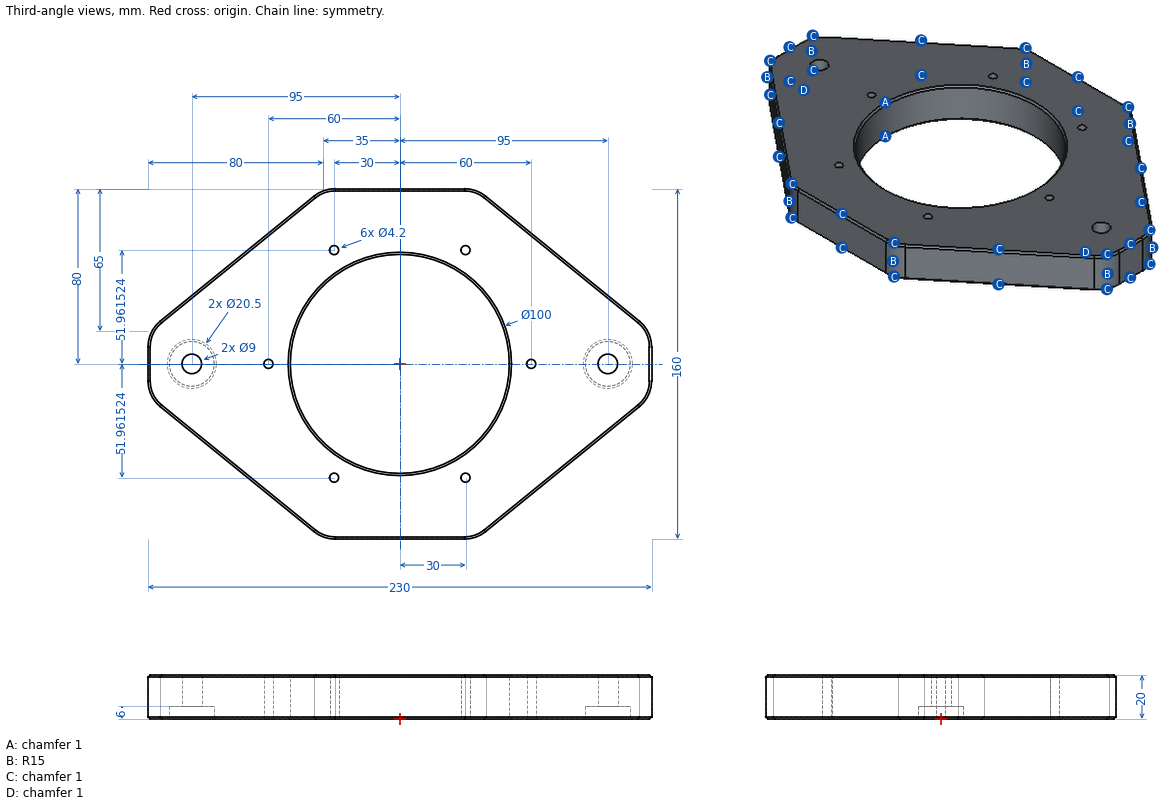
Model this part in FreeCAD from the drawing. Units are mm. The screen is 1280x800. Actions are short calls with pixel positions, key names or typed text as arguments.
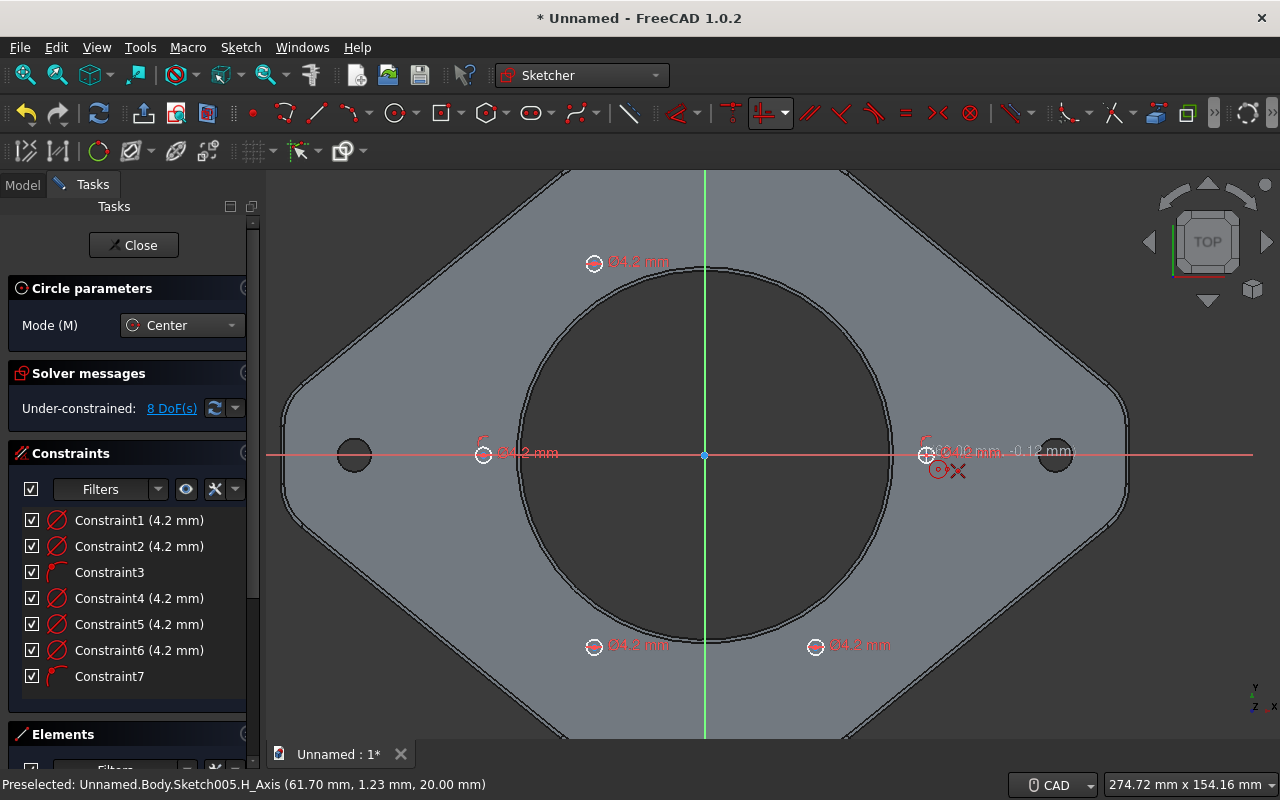
scroll(816, 263, up, 6)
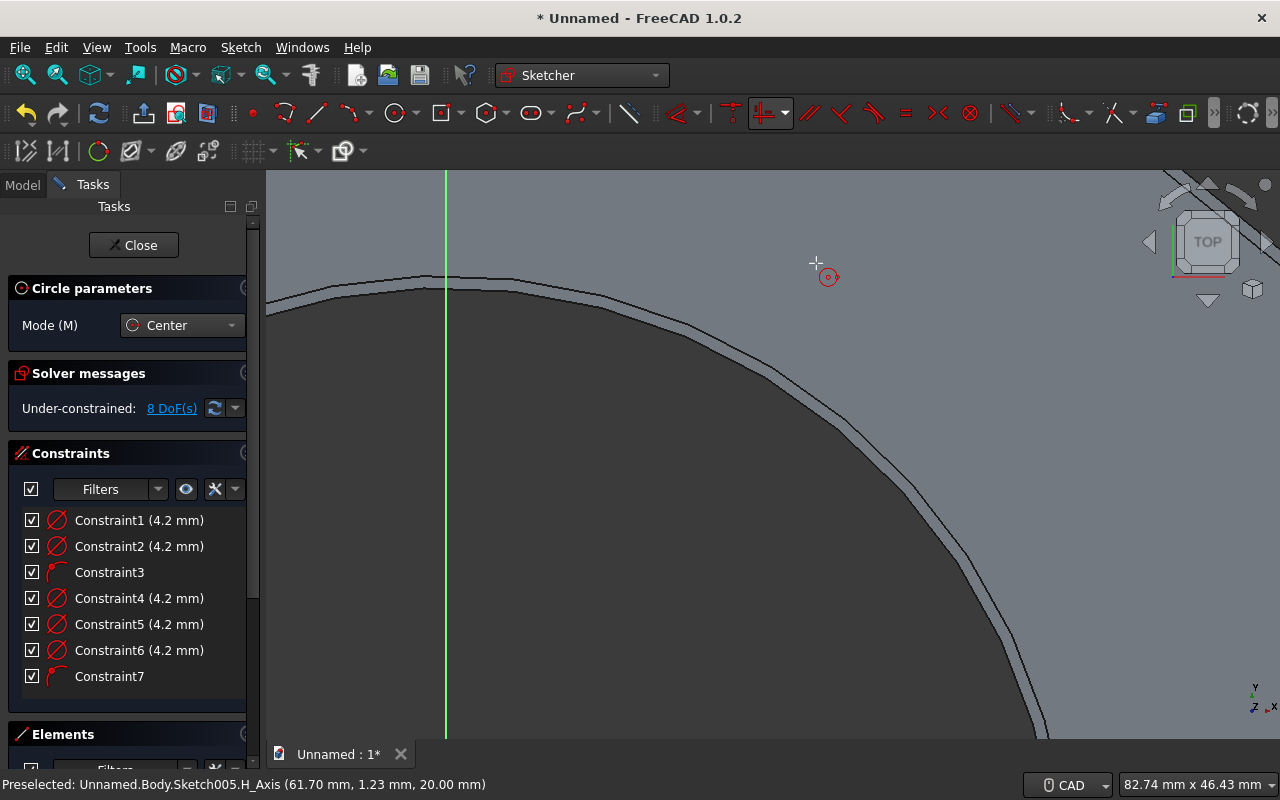
click(814, 264)
move(832, 246)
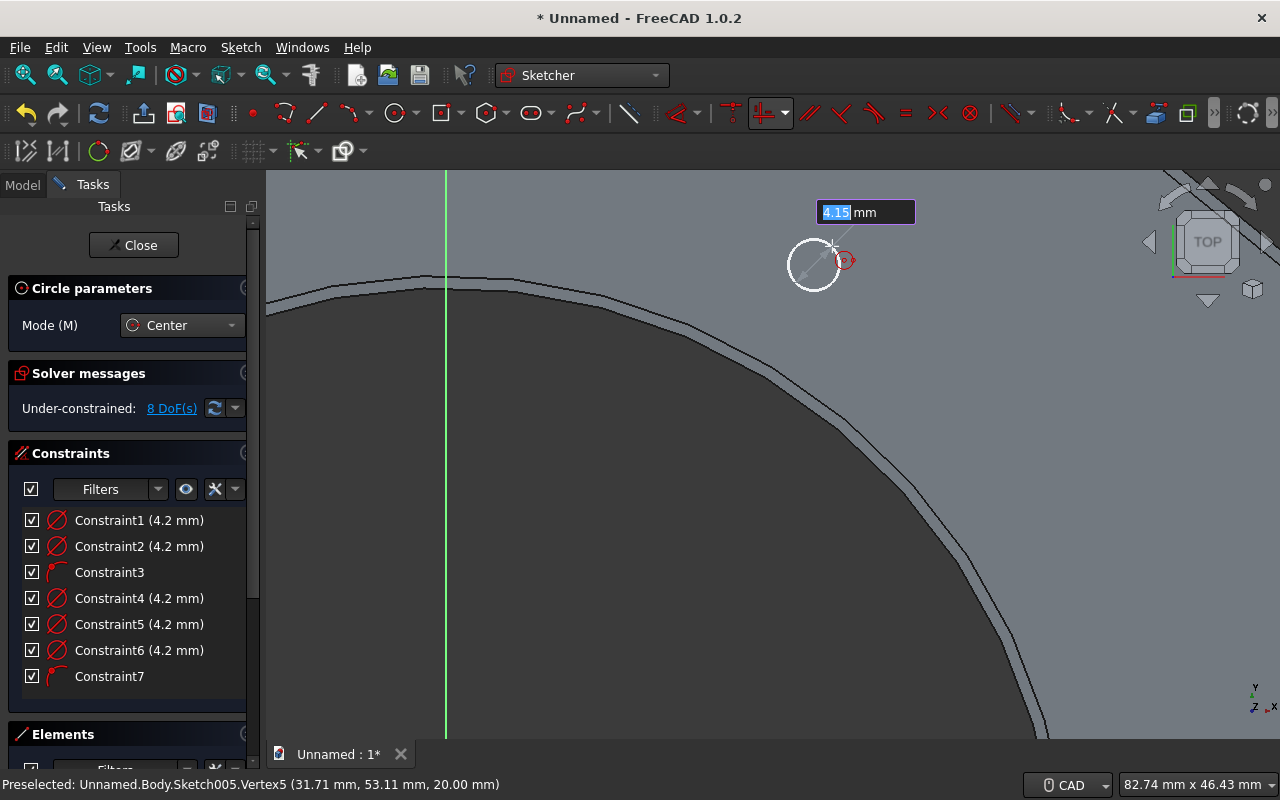
text(4.2)
key(Return)
key(Escape)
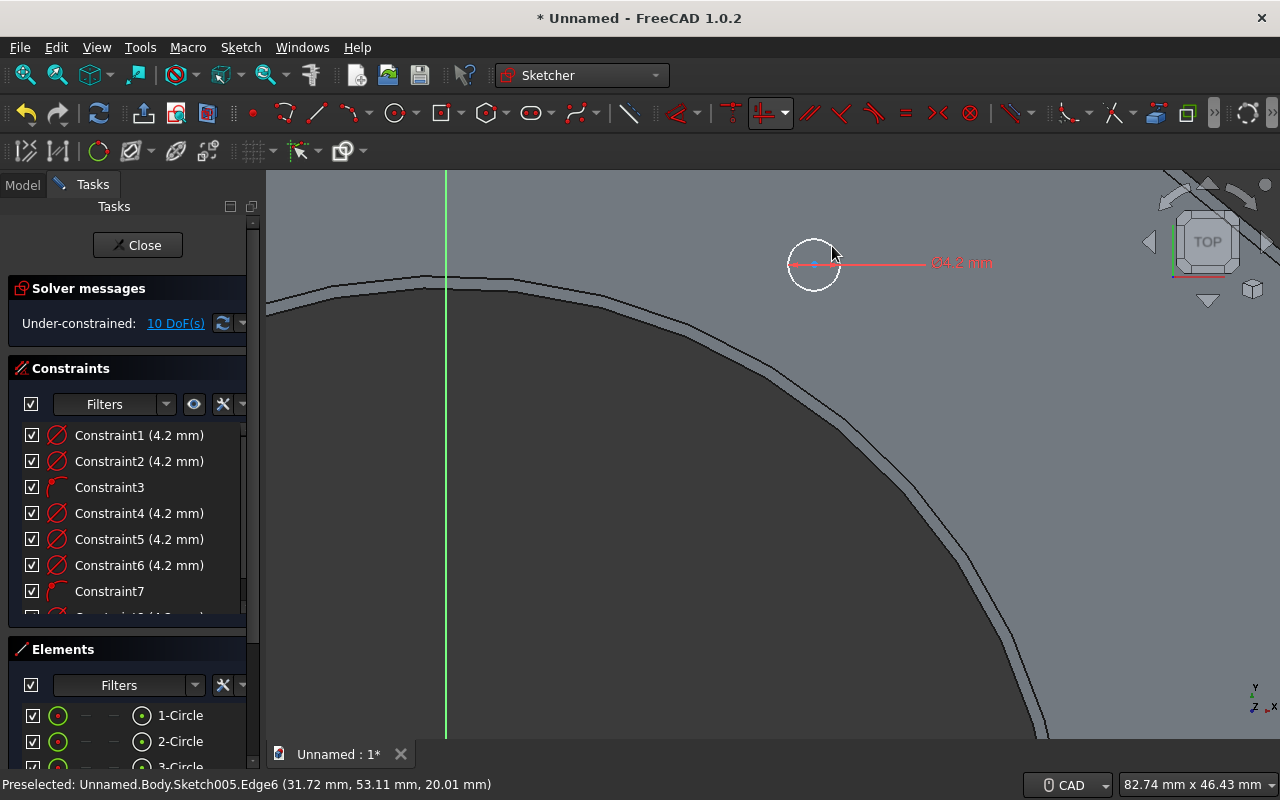
scroll(816, 262, down, 6)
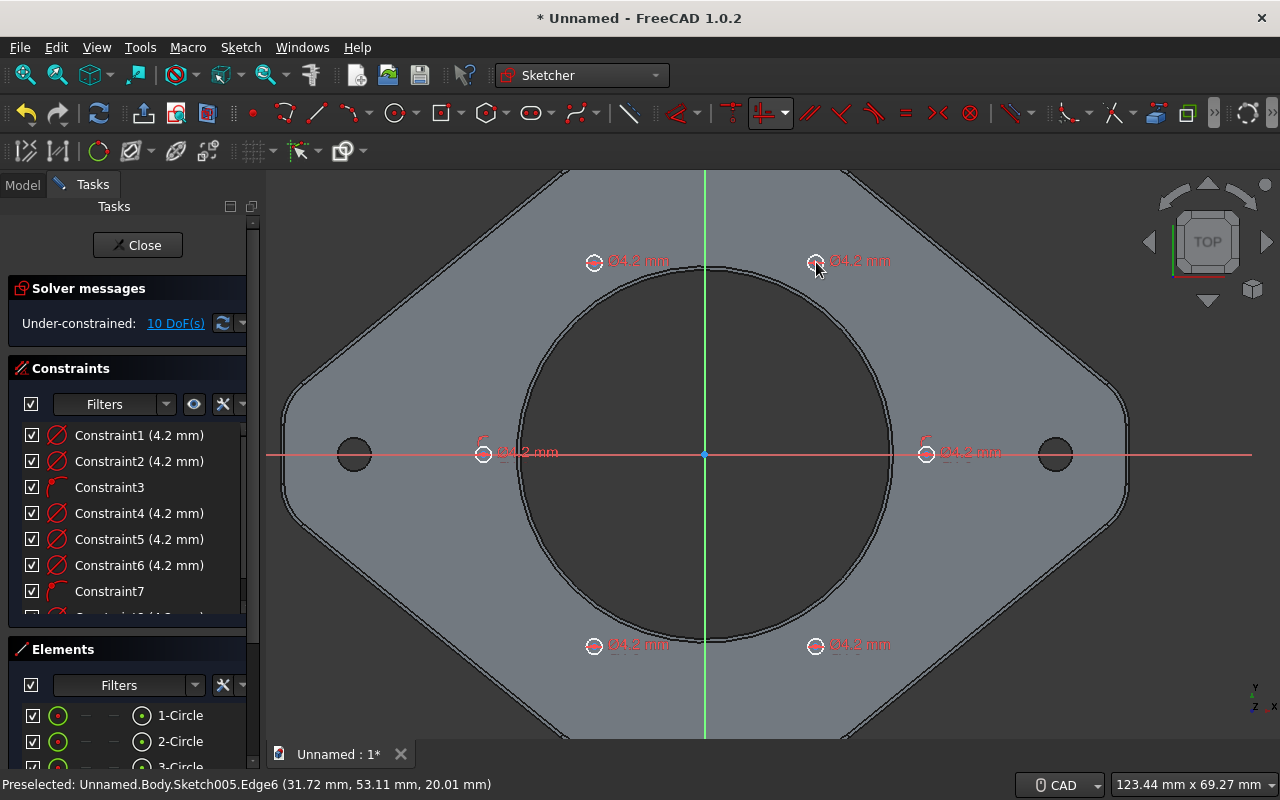
click(594, 263)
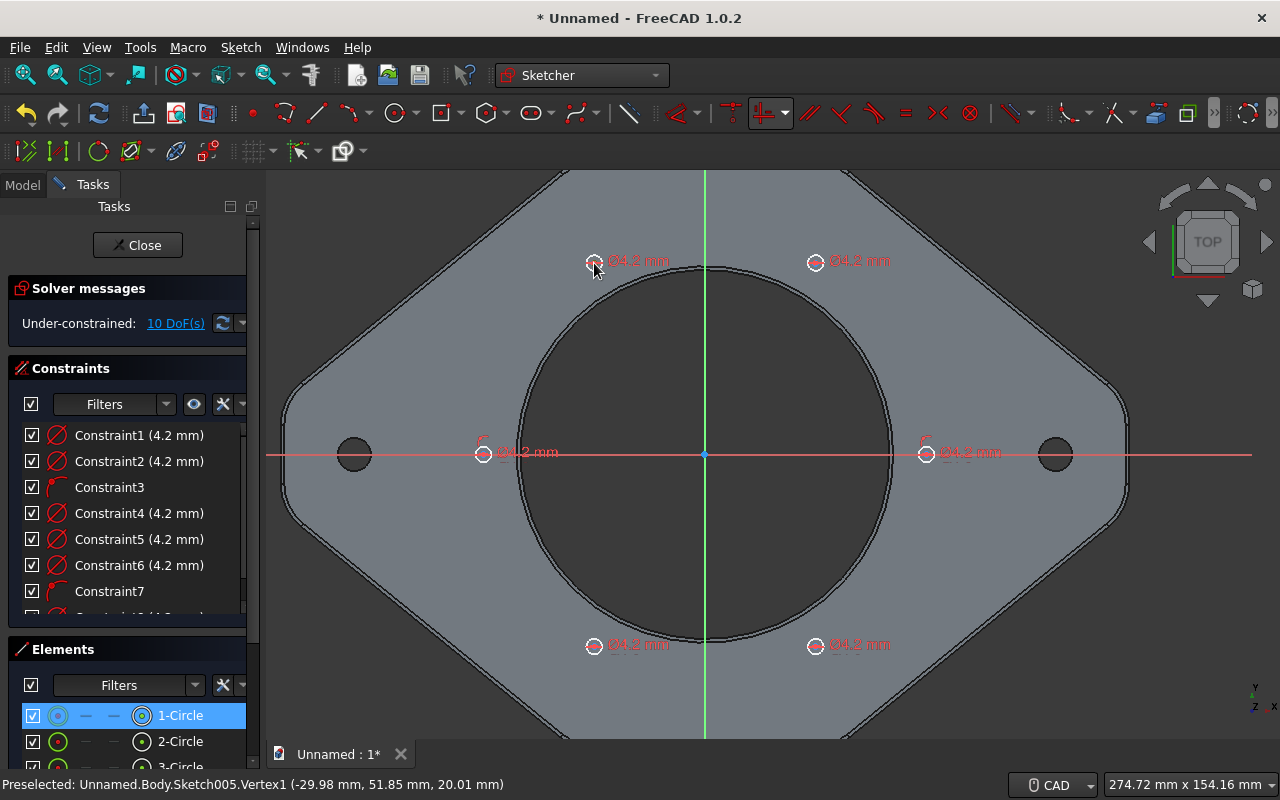
click(594, 647)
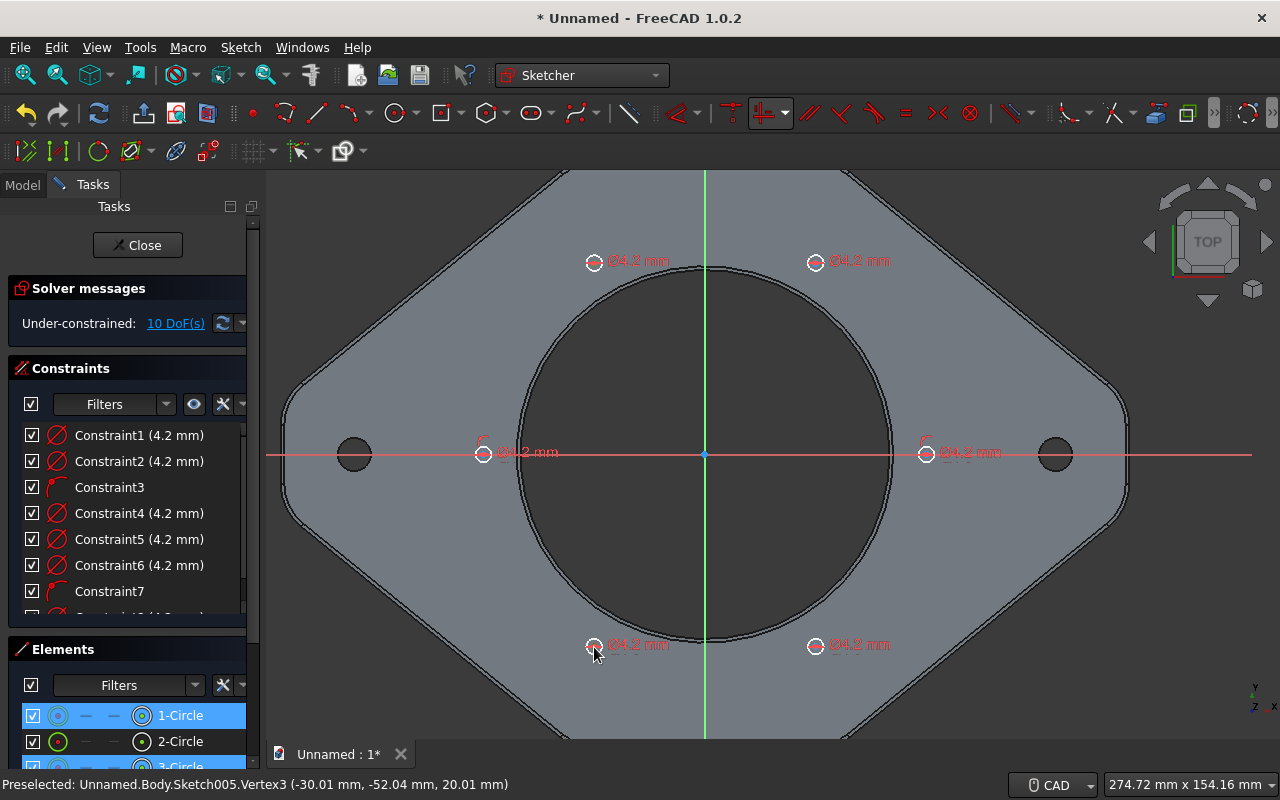
click(788, 114)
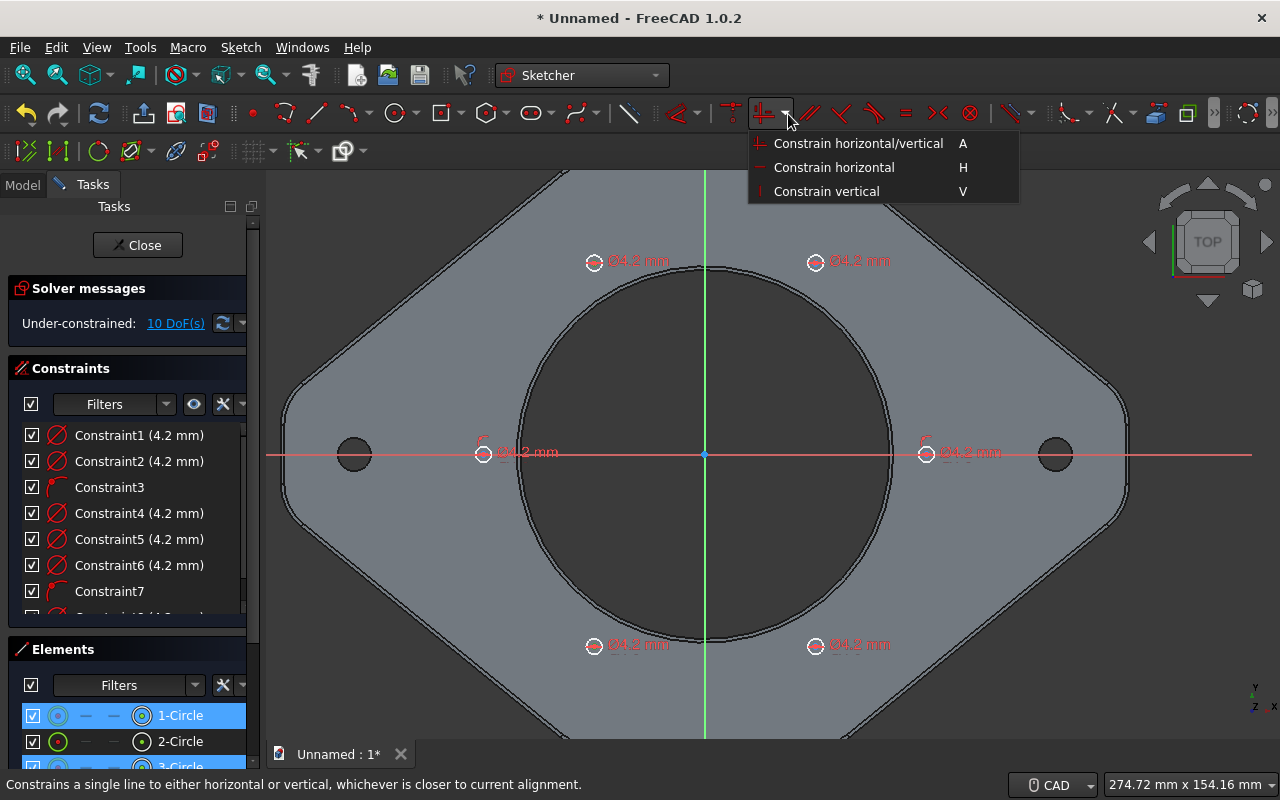
click(884, 191)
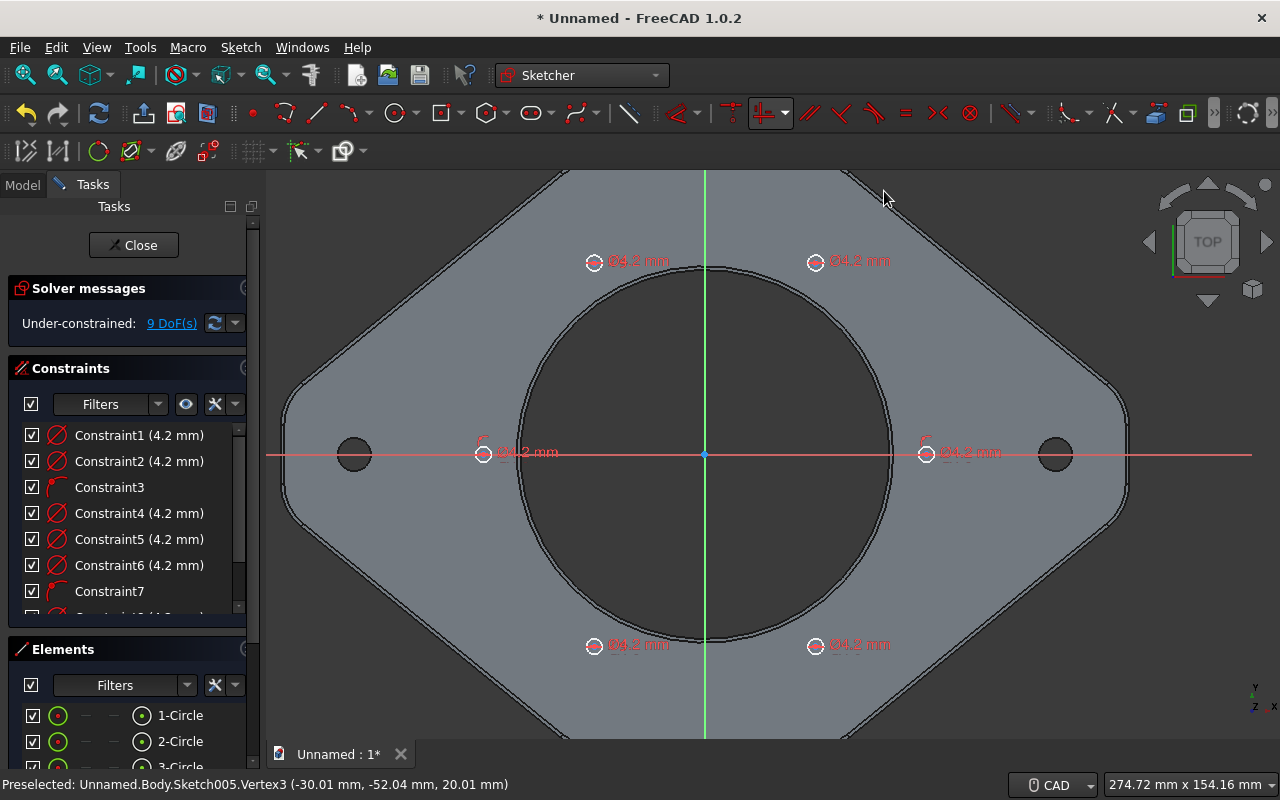
click(594, 647)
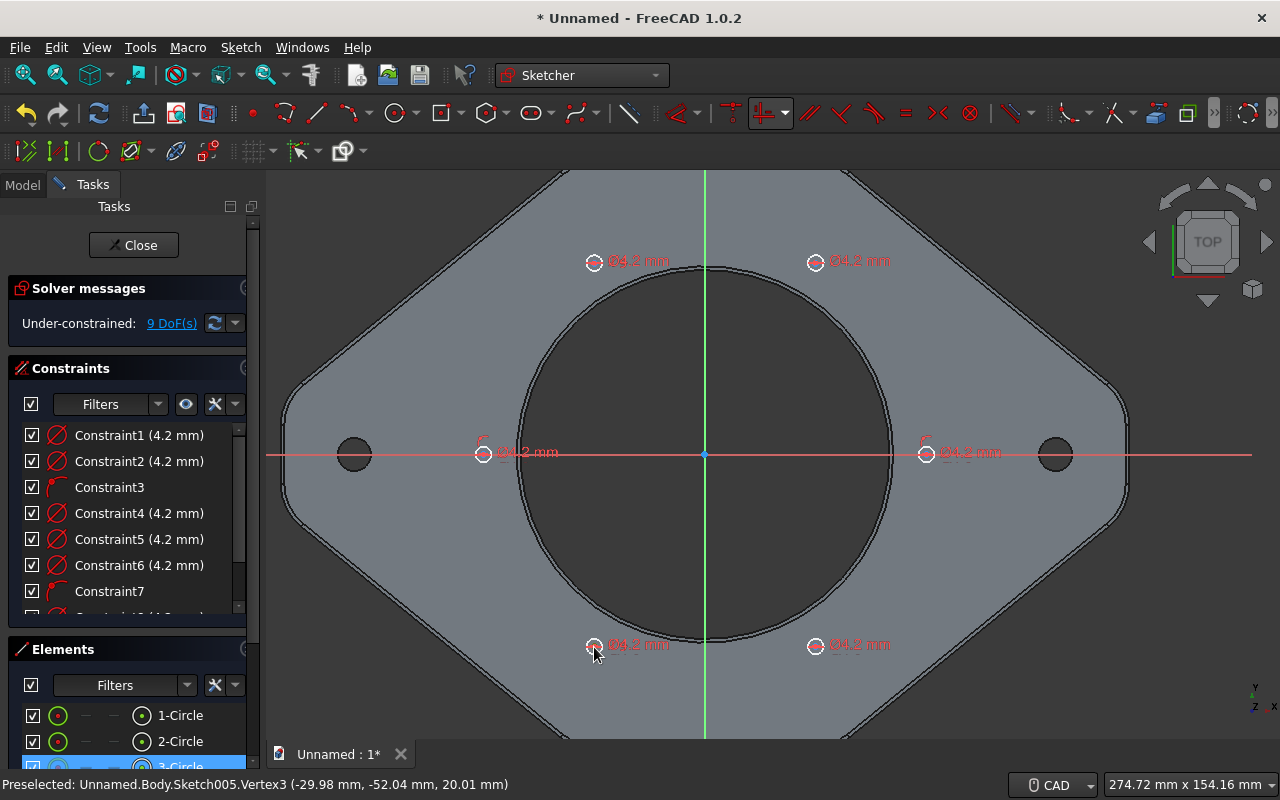
click(816, 647)